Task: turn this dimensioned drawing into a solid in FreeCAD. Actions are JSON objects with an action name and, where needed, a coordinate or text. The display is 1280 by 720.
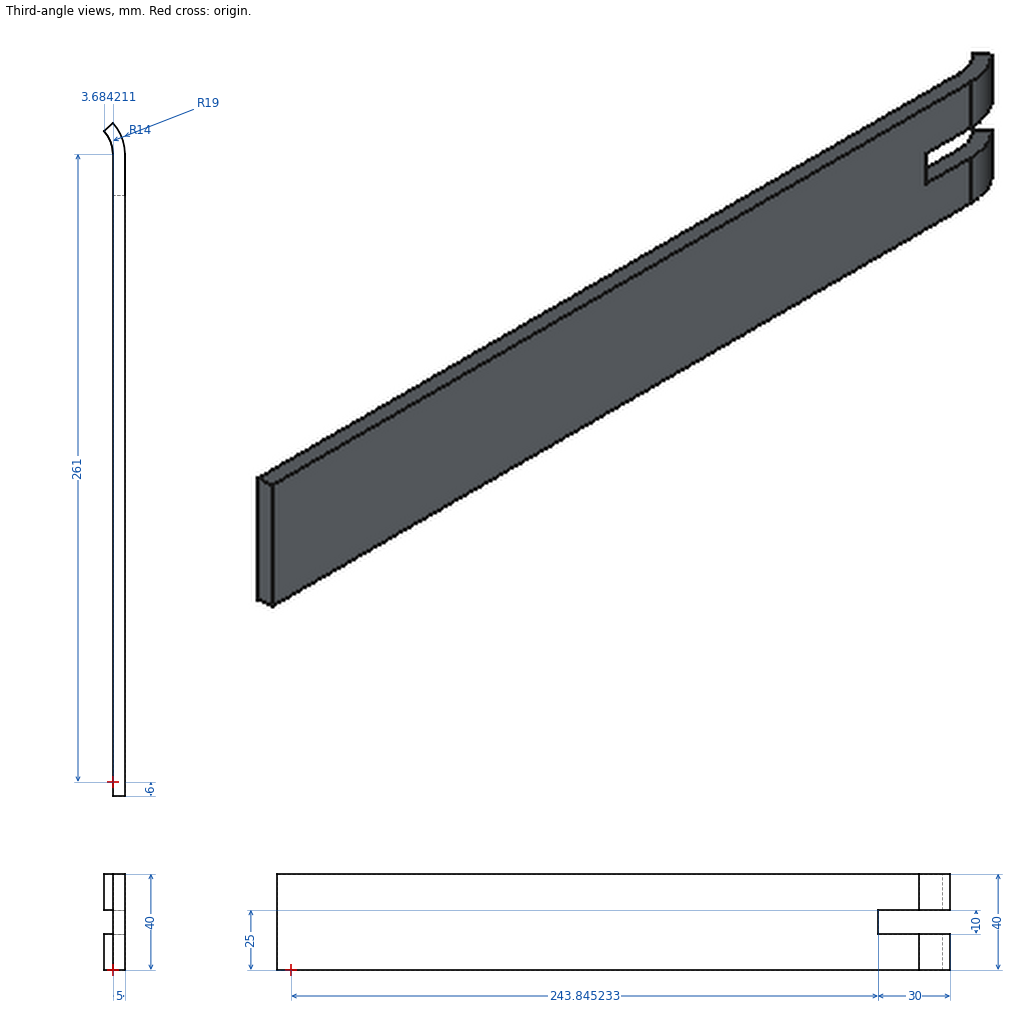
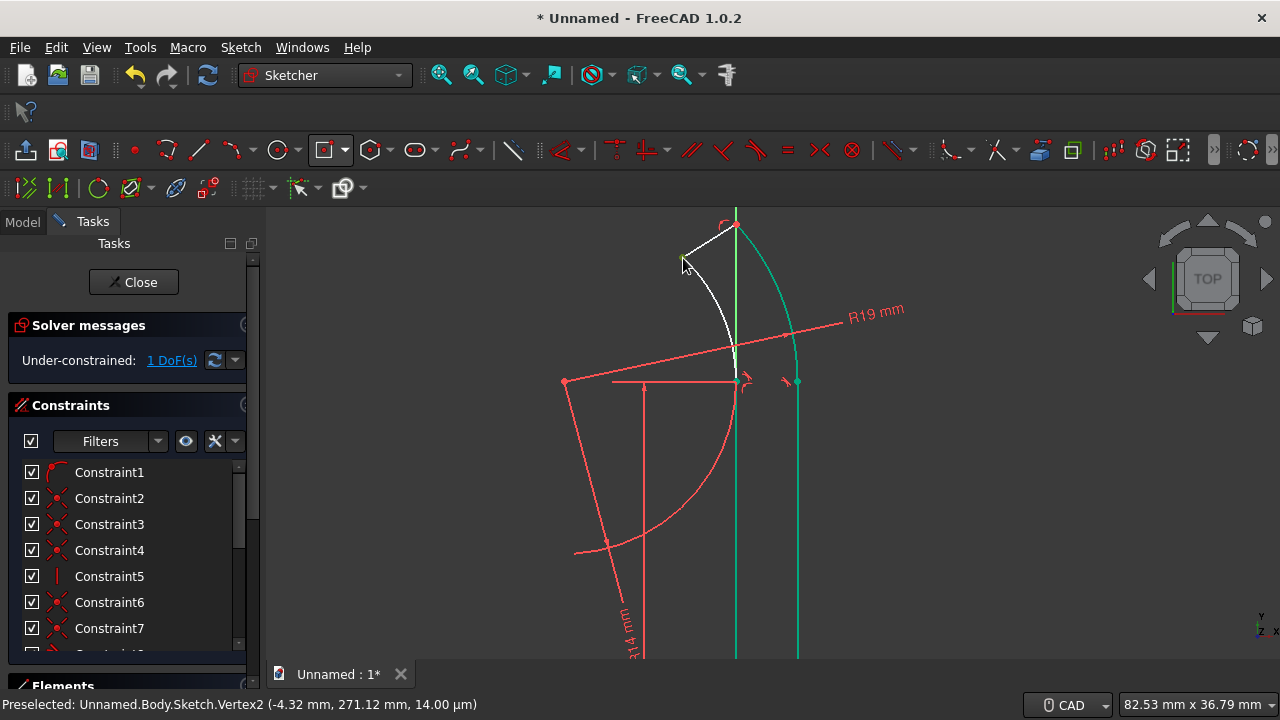
{"action": "left_click", "coordinate": [584, 150]}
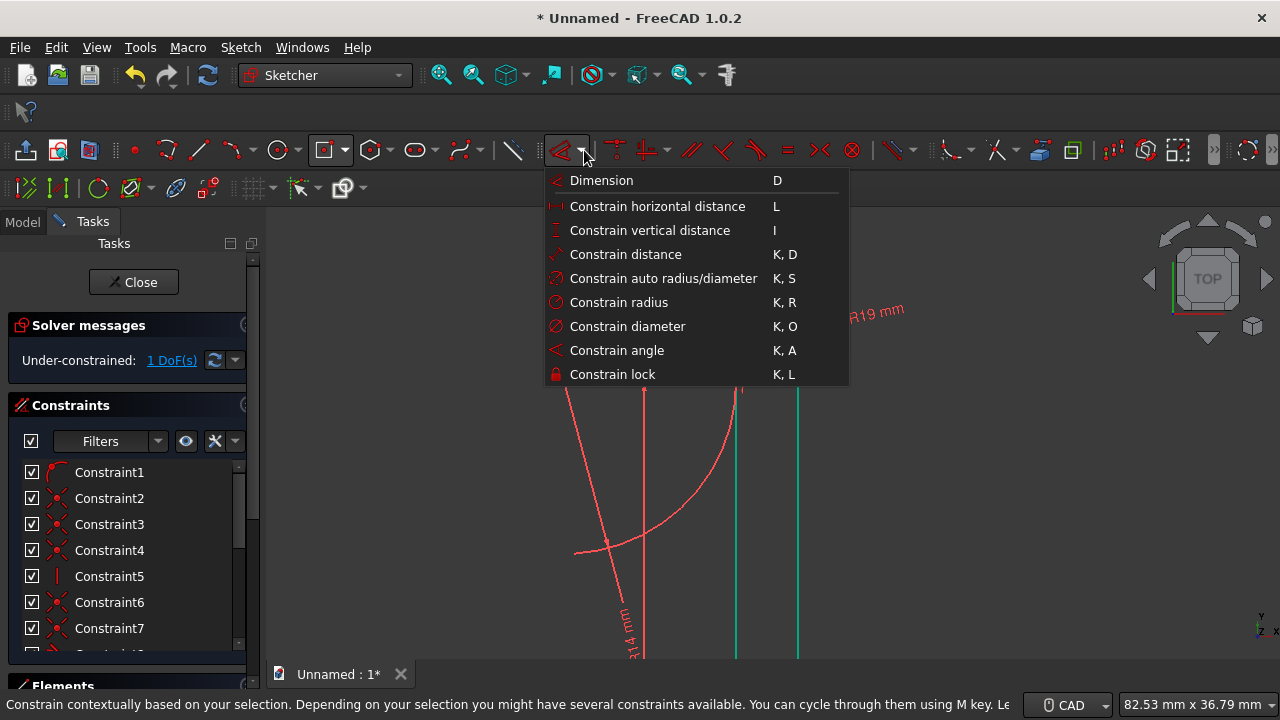
{"action": "left_click", "coordinate": [697, 206]}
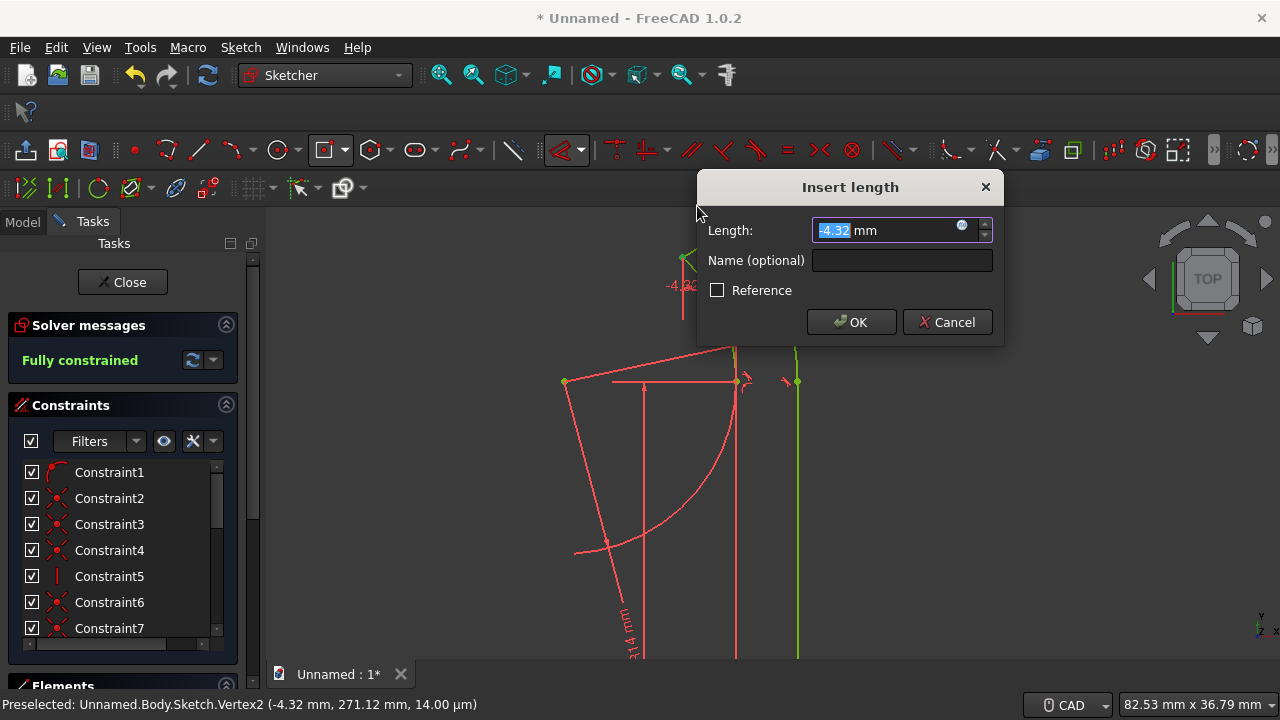
{"action": "type", "text": "-3.684211"}
{"action": "key", "text": "Return"}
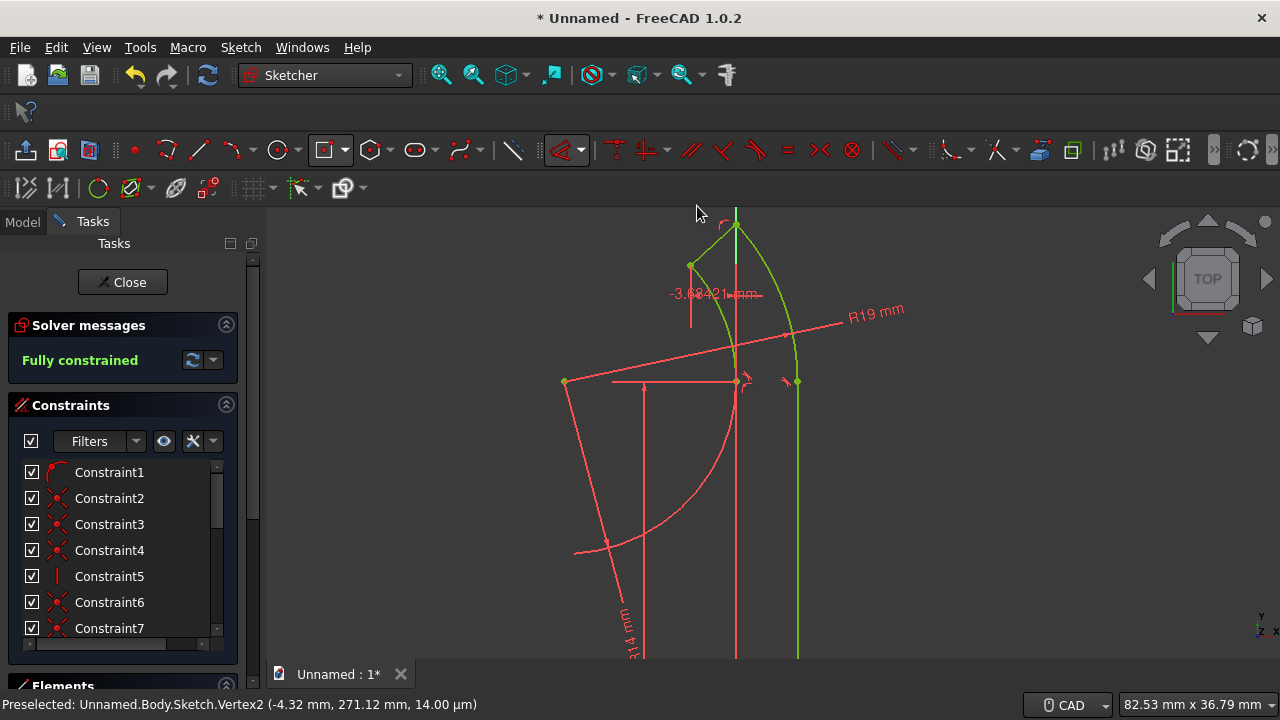
{"action": "left_click", "coordinate": [123, 282]}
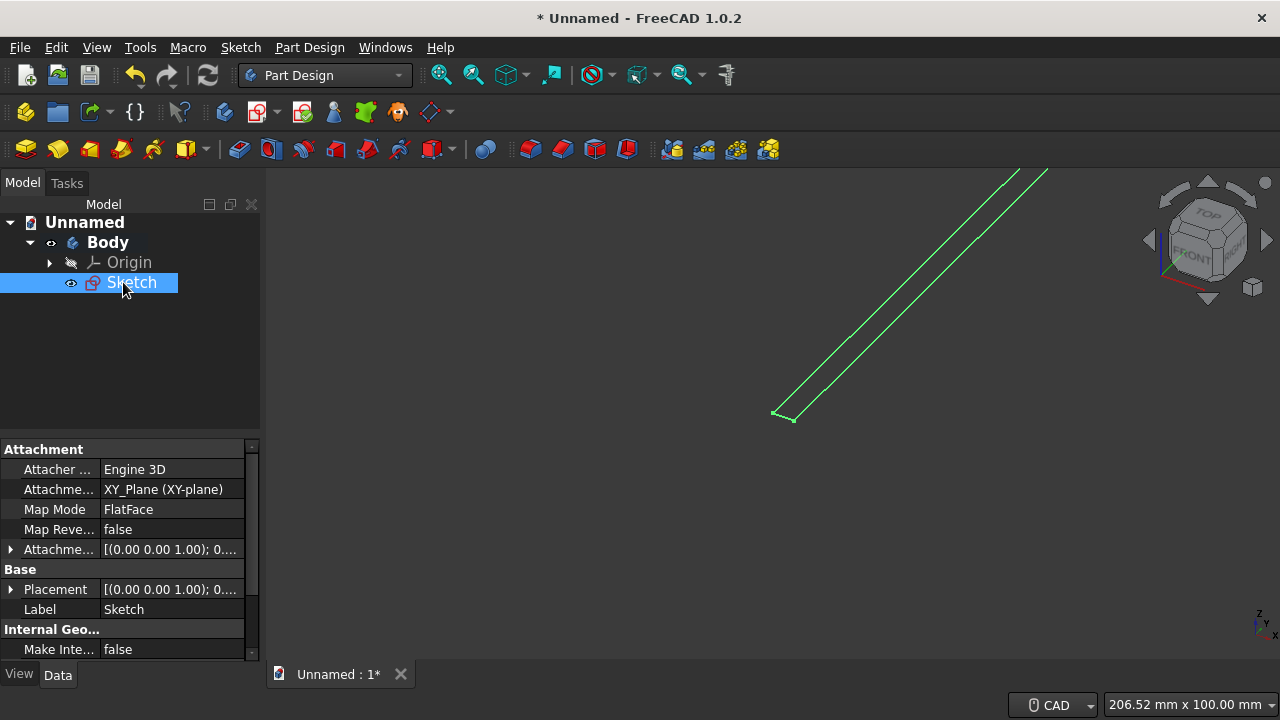
{"action": "left_click", "coordinate": [26, 150]}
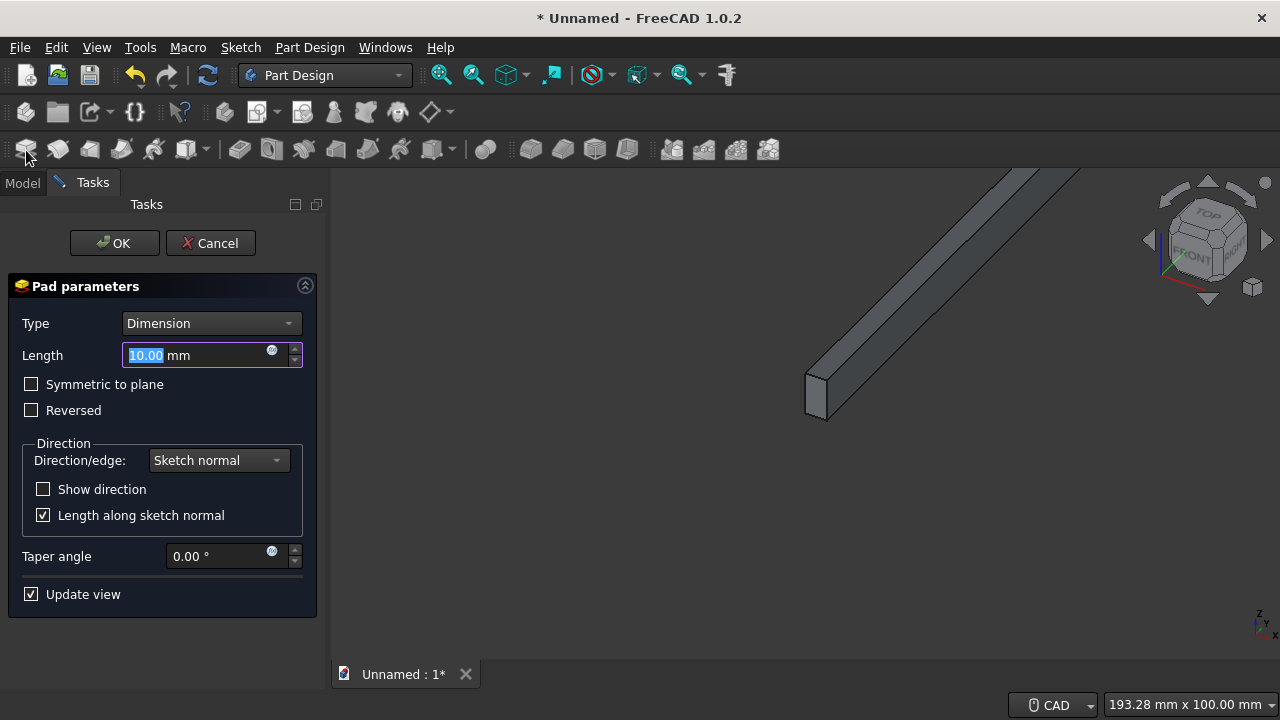
{"action": "type", "text": "40"}
{"action": "key", "text": "Tab"}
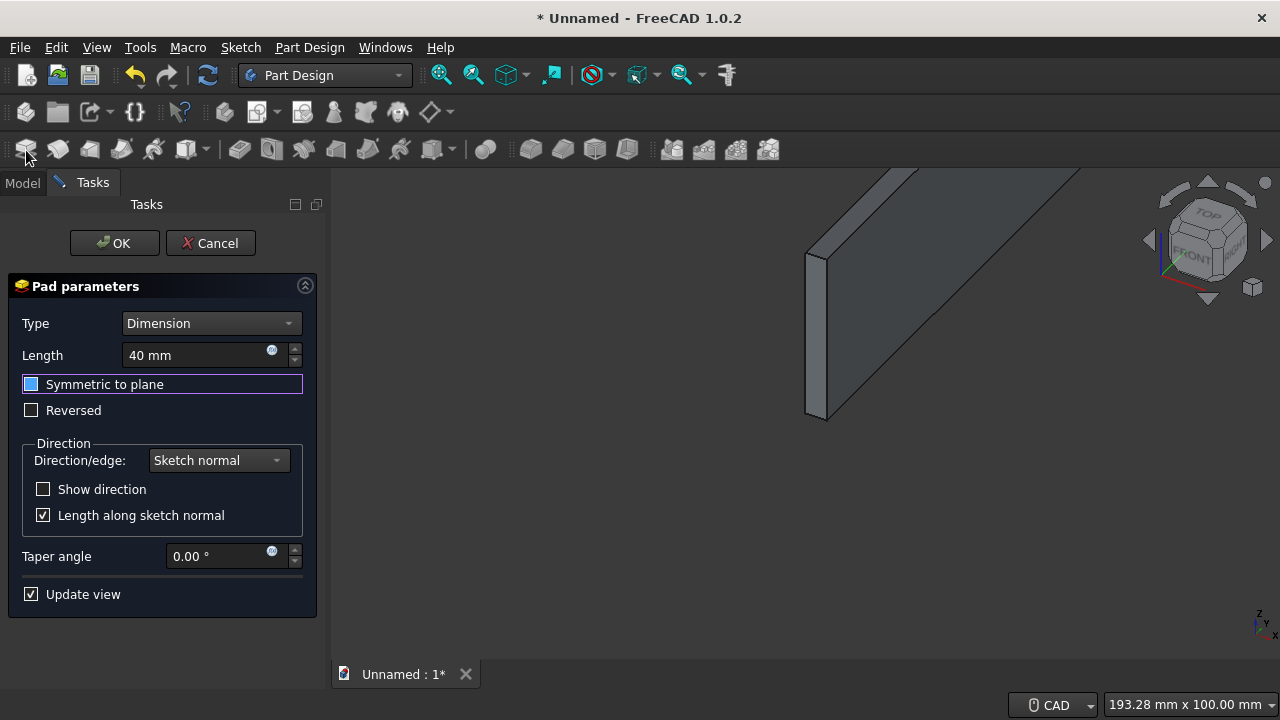
{"action": "left_click", "coordinate": [115, 243]}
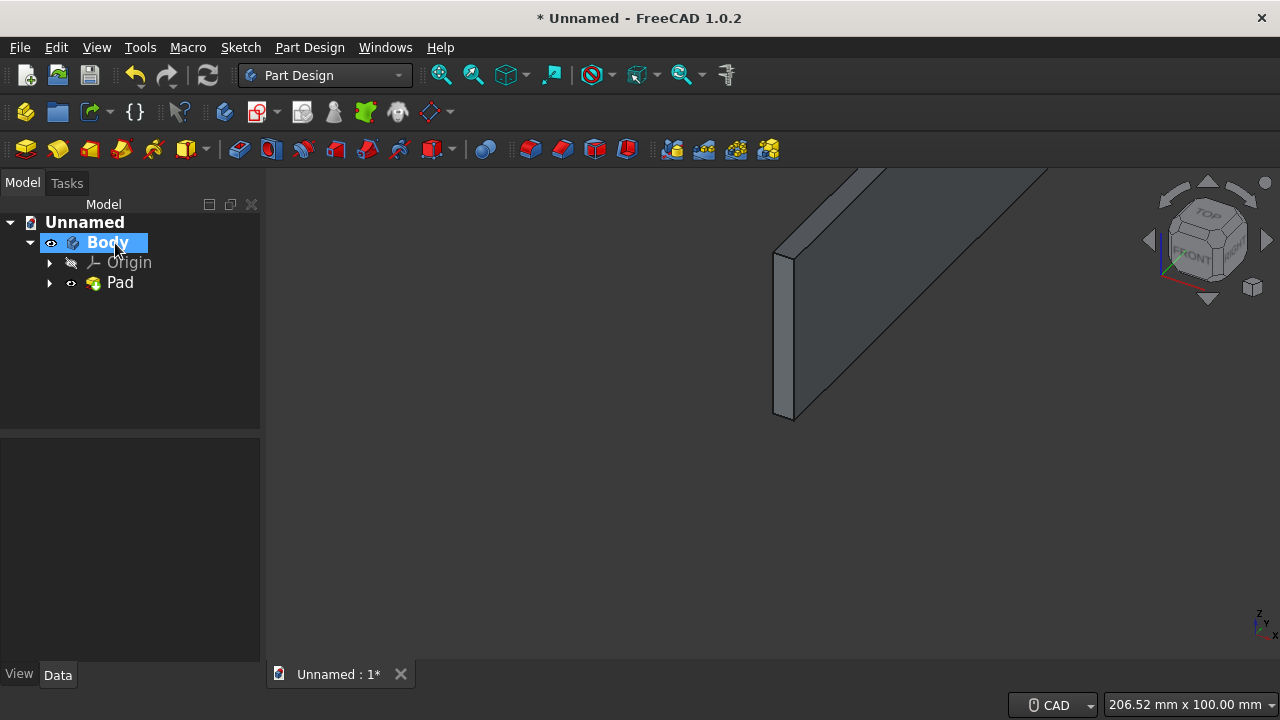
{"action": "key", "text": "v f"}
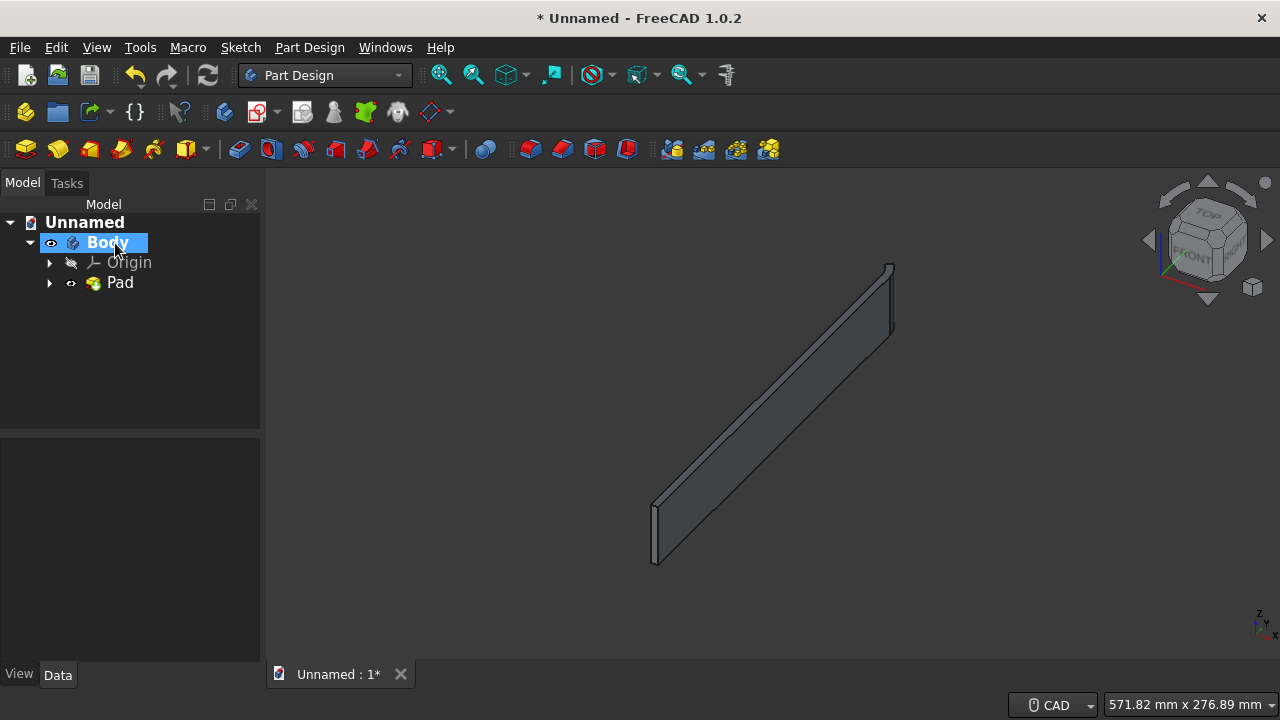
{"action": "left_click", "coordinate": [840, 355]}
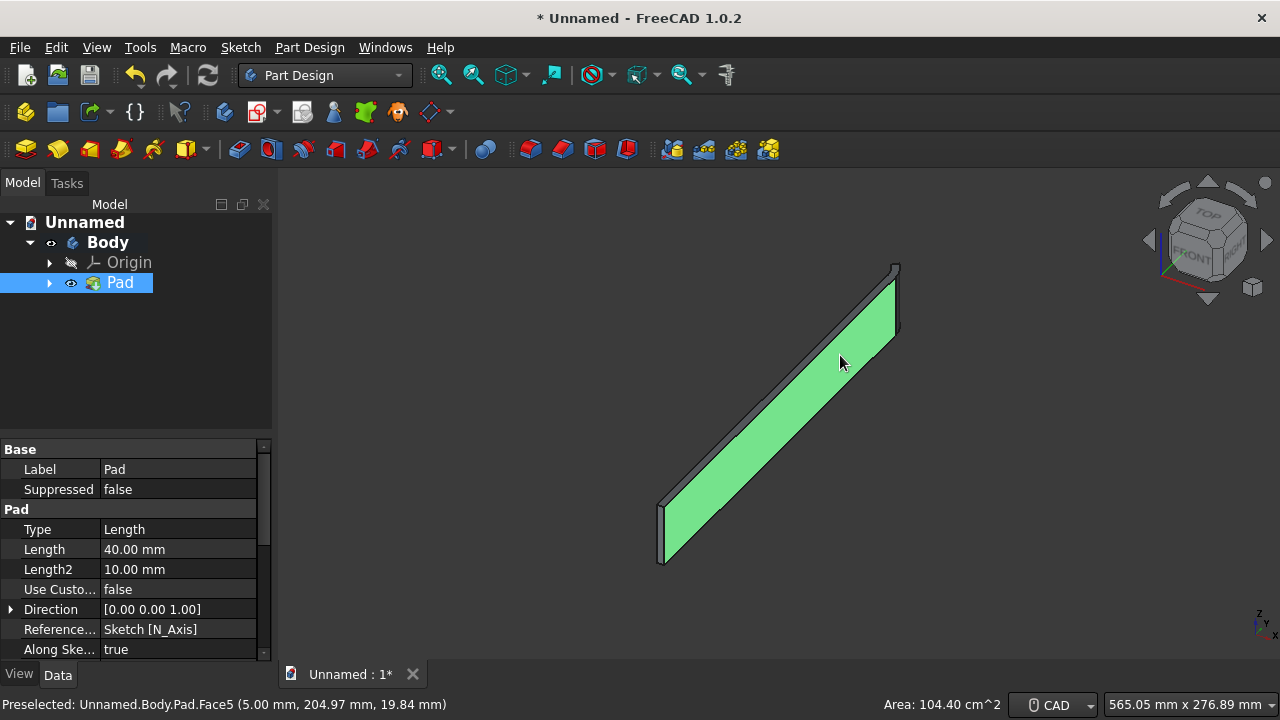
{"action": "left_click", "coordinate": [258, 112]}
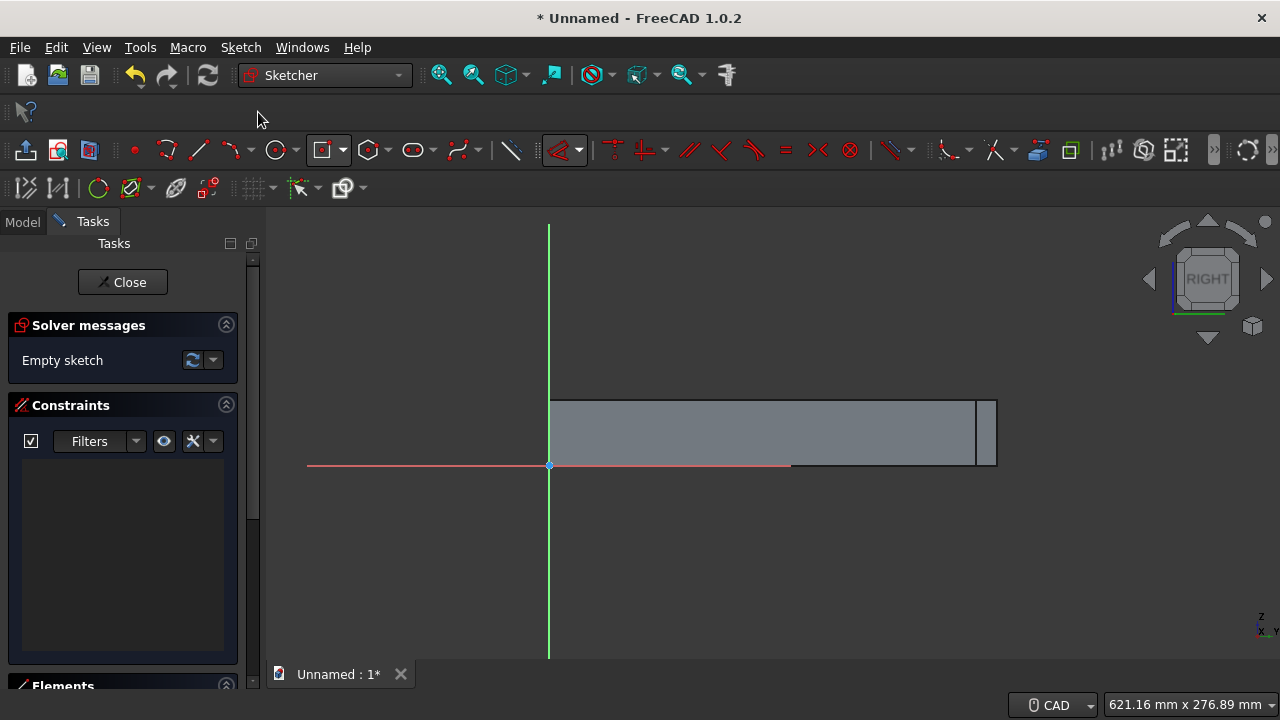
{"action": "scroll", "coordinate": [999, 433], "scroll_direction": "up", "scroll_amount": 12}